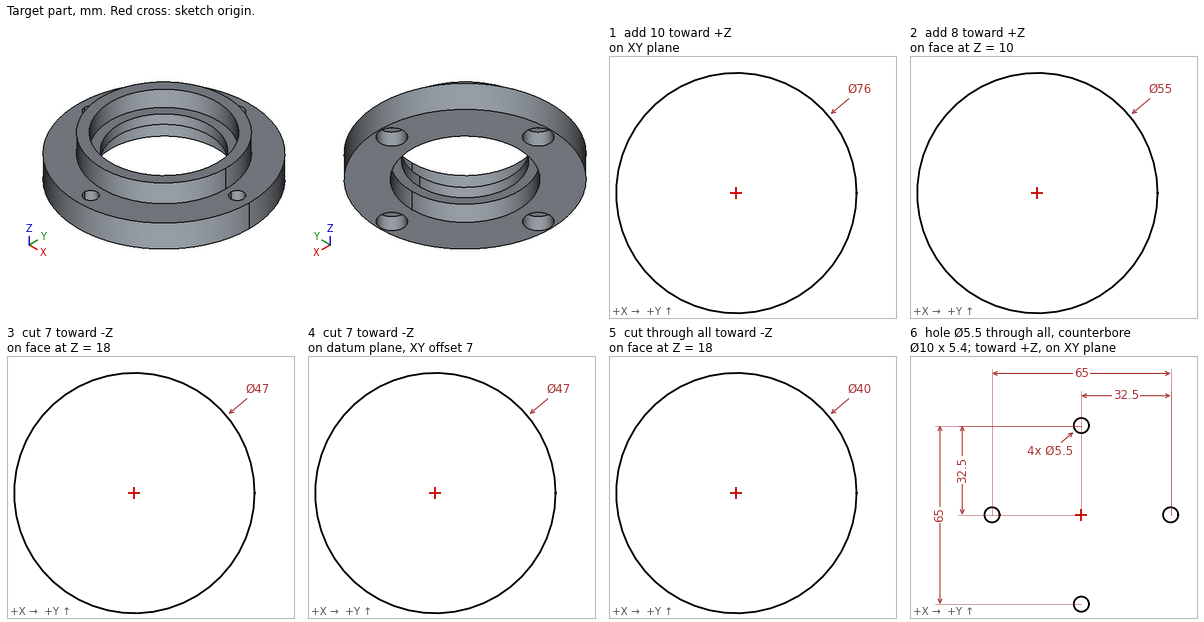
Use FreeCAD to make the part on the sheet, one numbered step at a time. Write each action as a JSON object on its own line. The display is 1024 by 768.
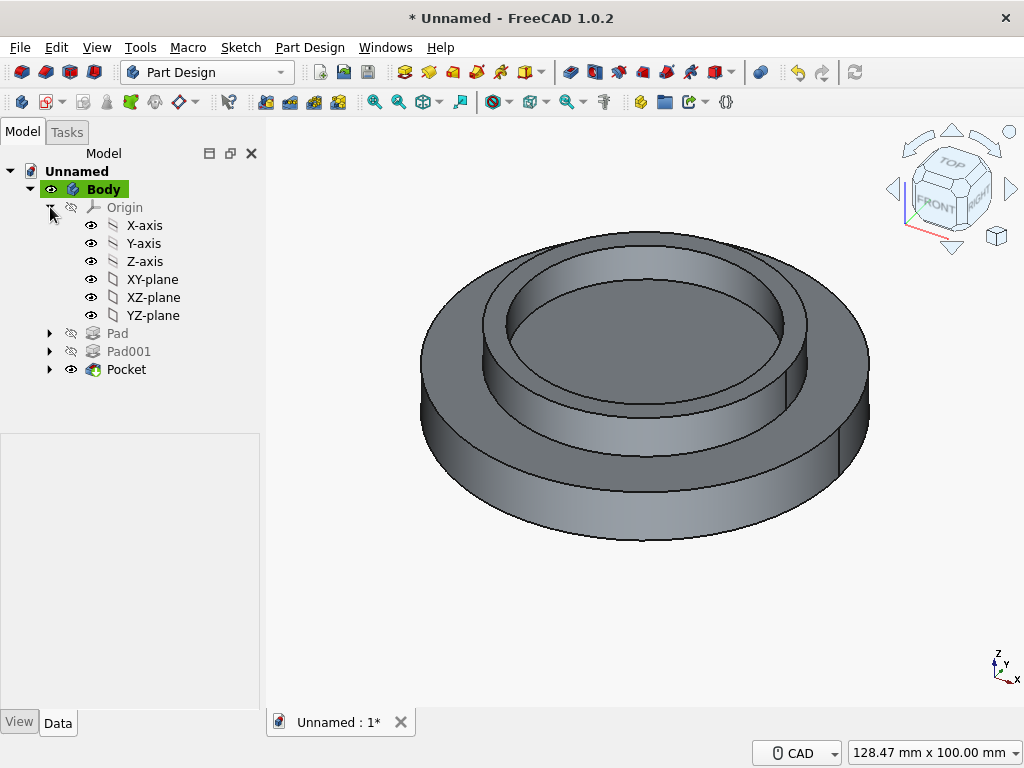
{"action": "left_click", "coordinate": [136, 279]}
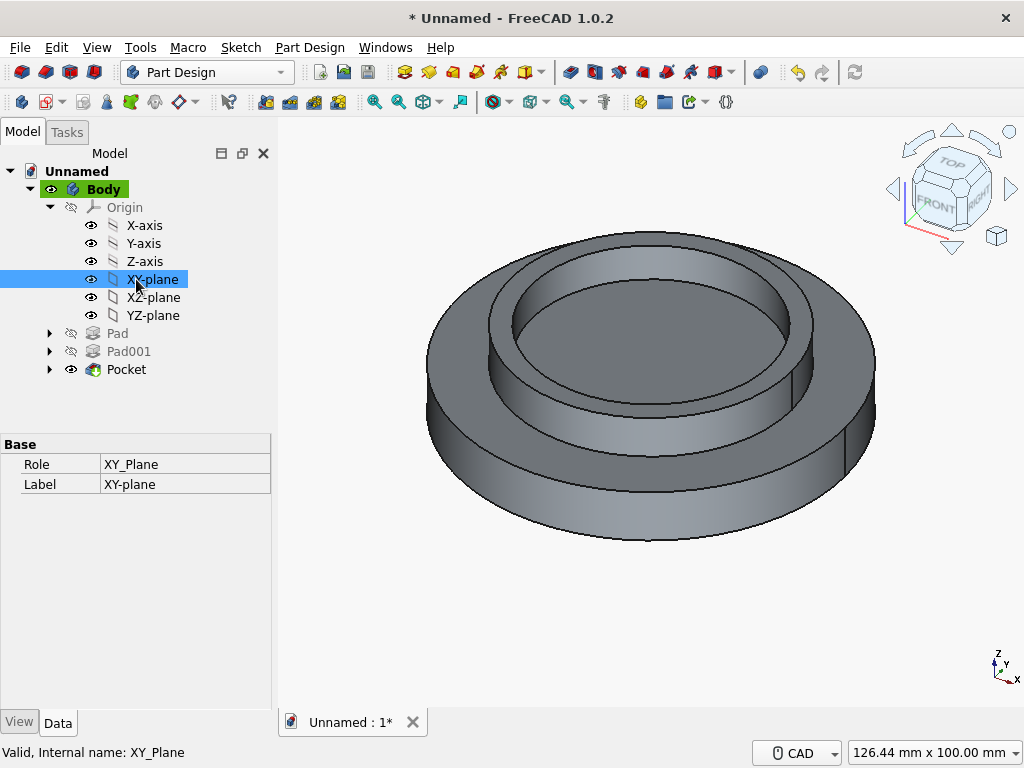
{"action": "left_click", "coordinate": [180, 102]}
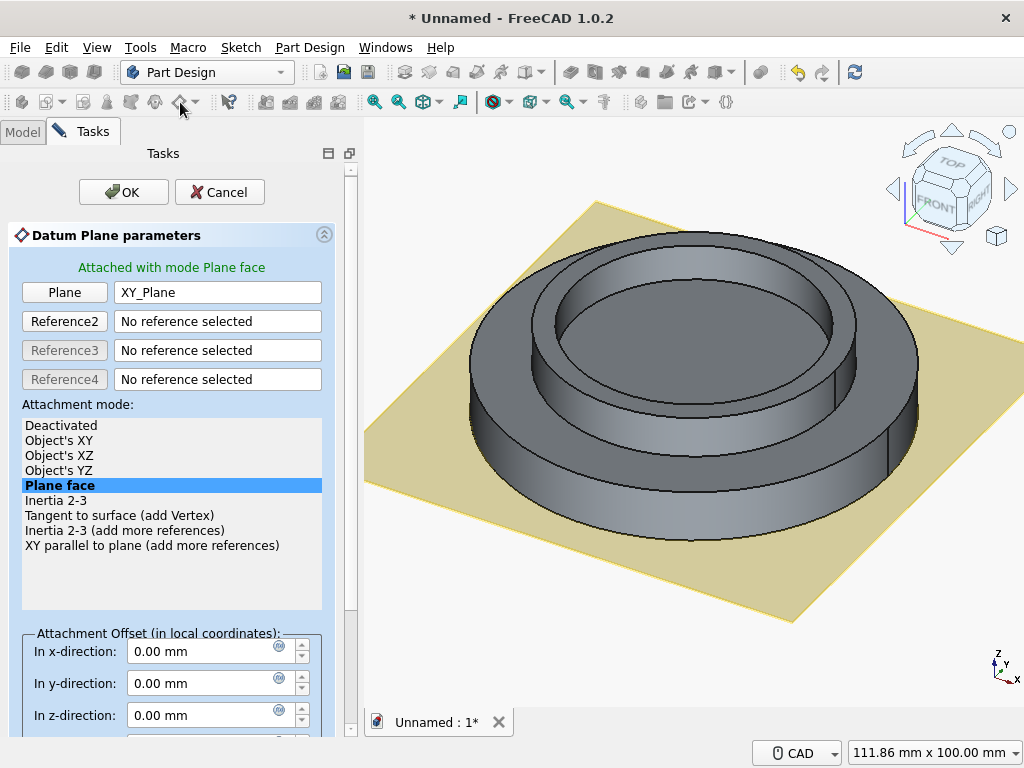
{"action": "triple_click", "coordinate": [210, 715]}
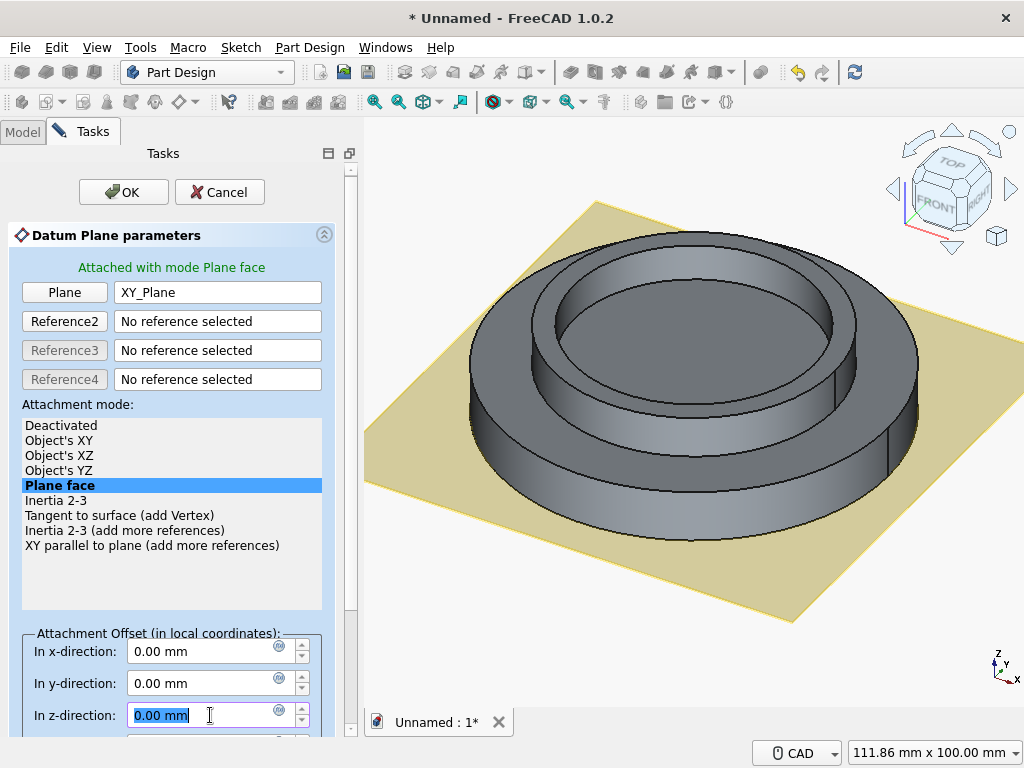
{"action": "type", "text": "7"}
{"action": "key", "text": "Tab"}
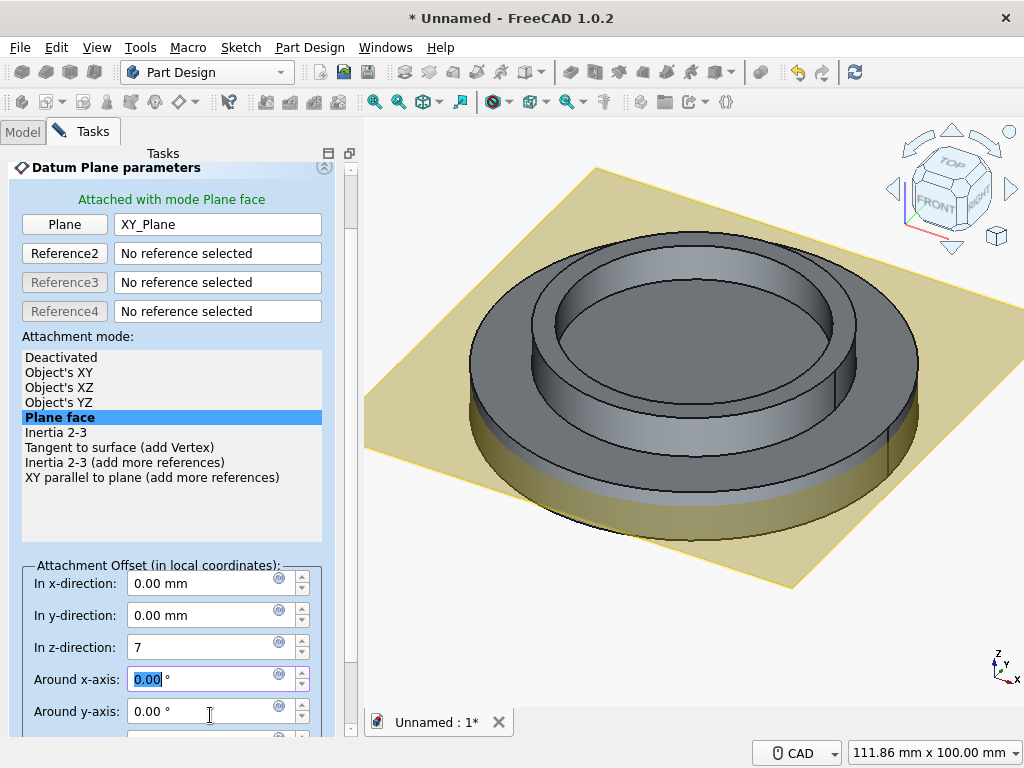
{"action": "scroll", "coordinate": [351, 450], "scroll_direction": "up", "scroll_amount": 2}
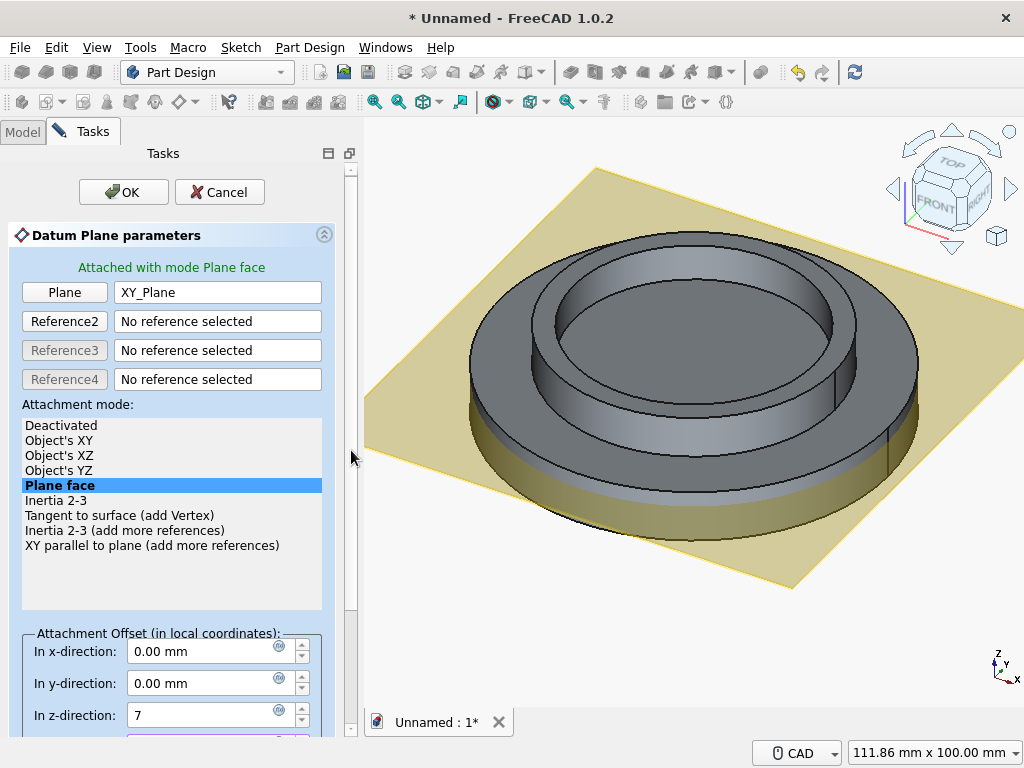
{"action": "left_click", "coordinate": [124, 192]}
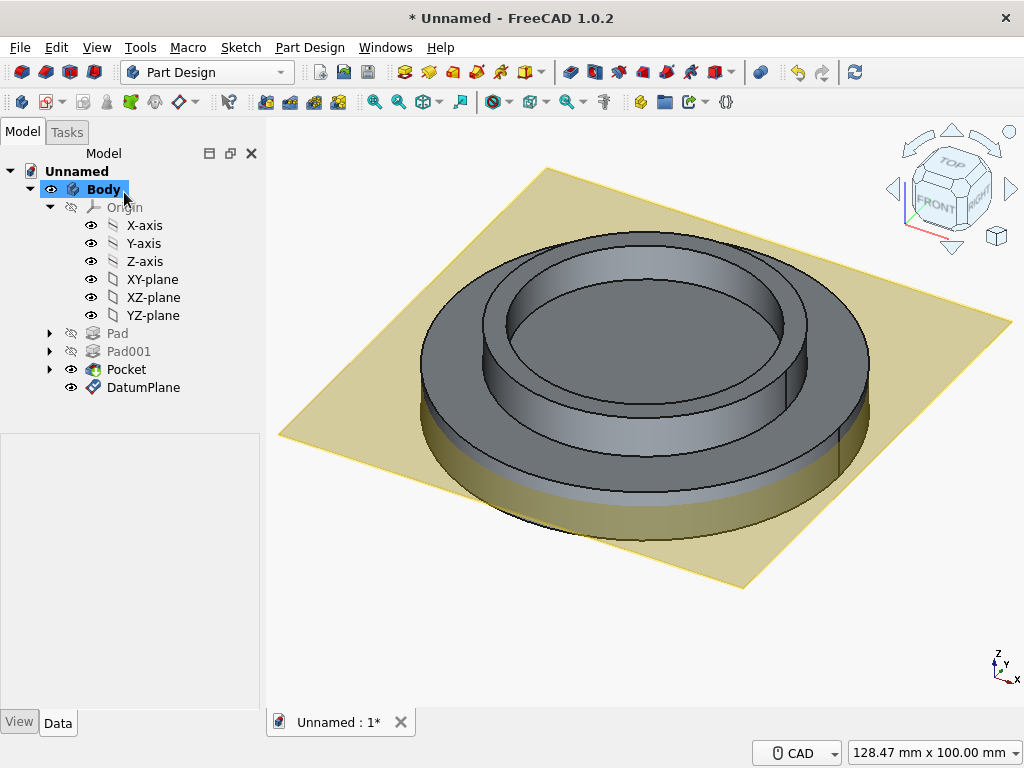
{"action": "left_click", "coordinate": [116, 387]}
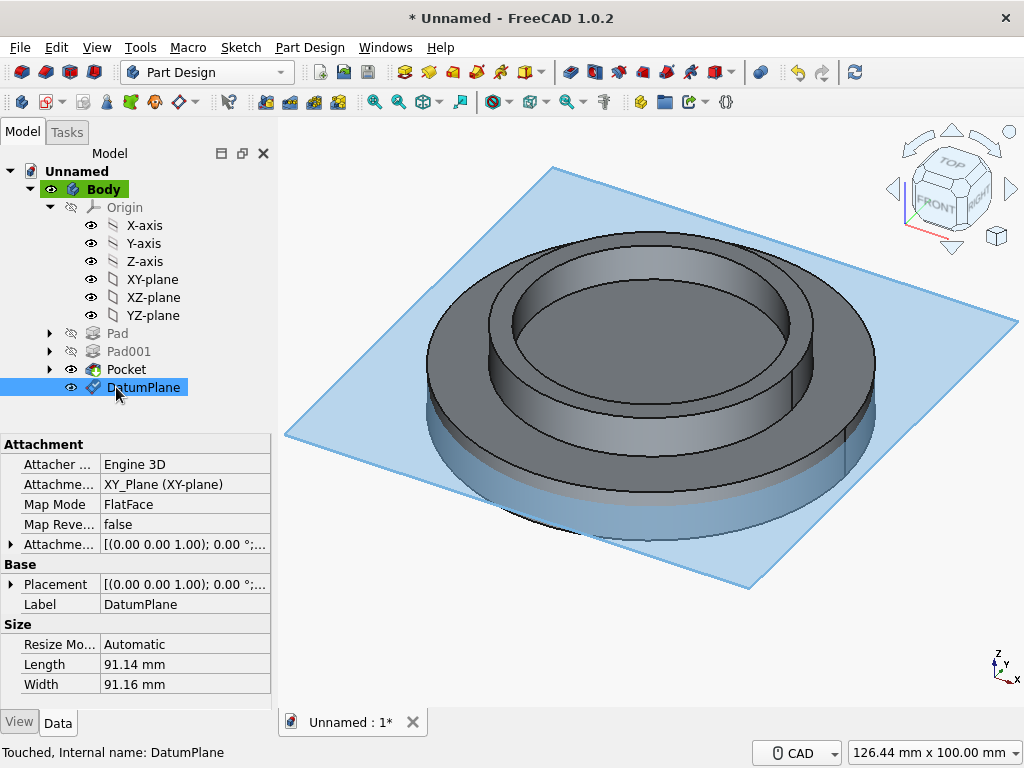
{"action": "left_click", "coordinate": [46, 102]}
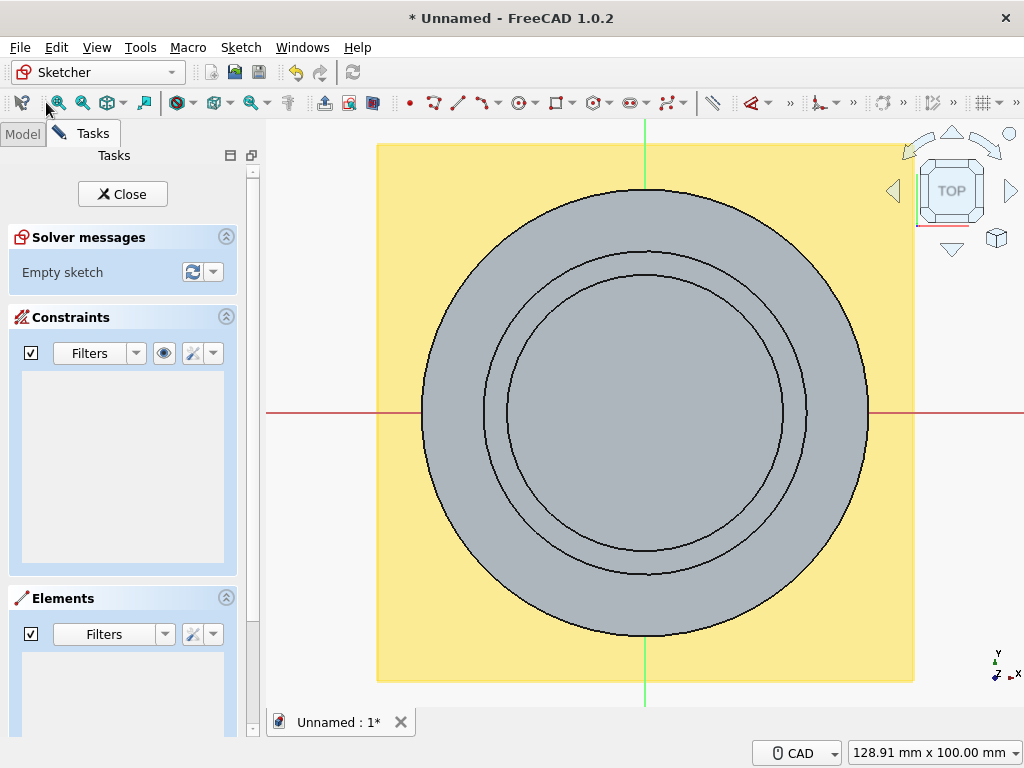
{"action": "left_click", "coordinate": [374, 104]}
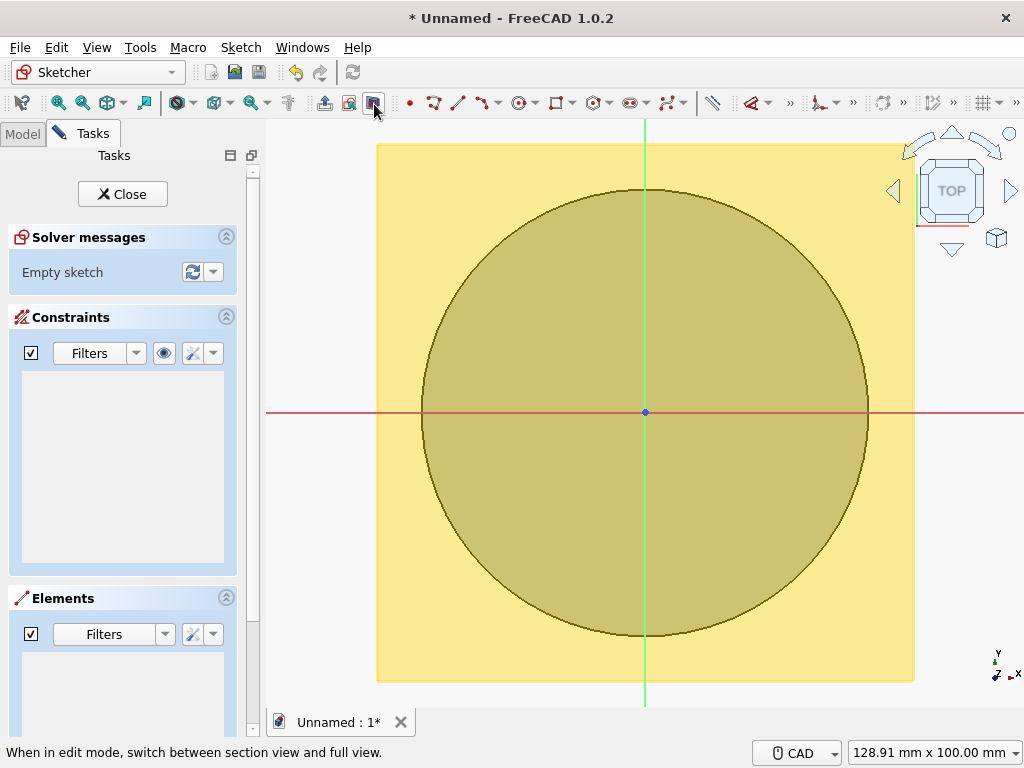
{"action": "scroll", "coordinate": [784, 413], "scroll_direction": "up", "scroll_amount": 2}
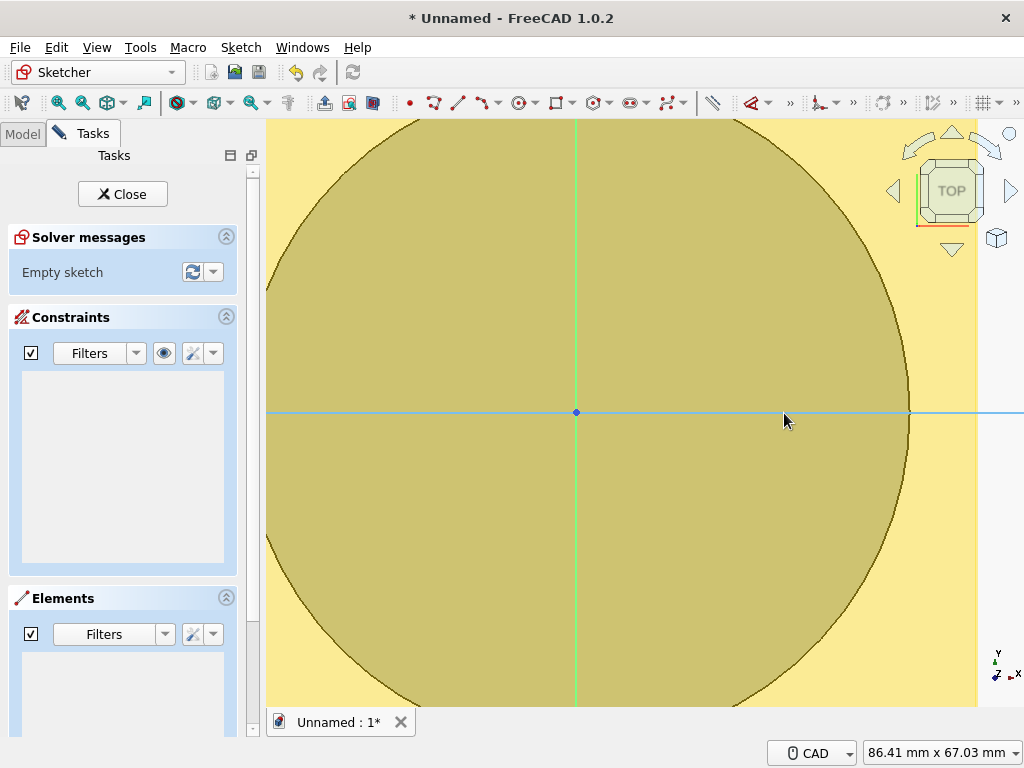
{"action": "key", "text": "g c"}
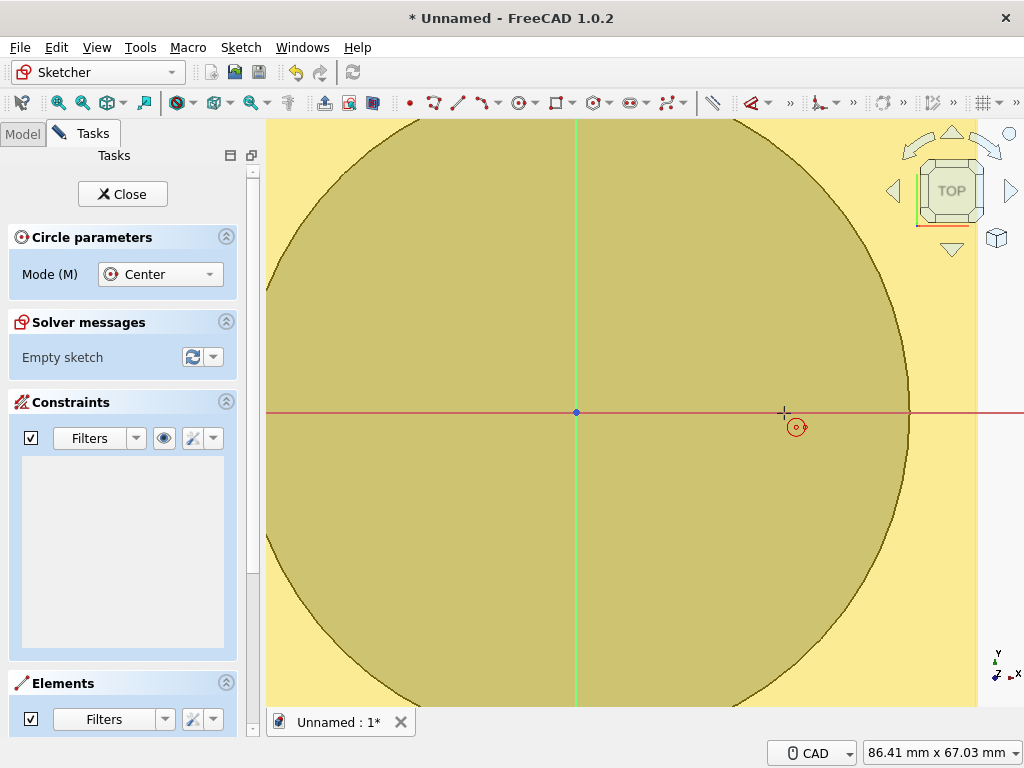
{"action": "left_click", "coordinate": [576, 413]}
{"action": "left_click", "coordinate": [722, 267]}
{"action": "key", "text": "Escape"}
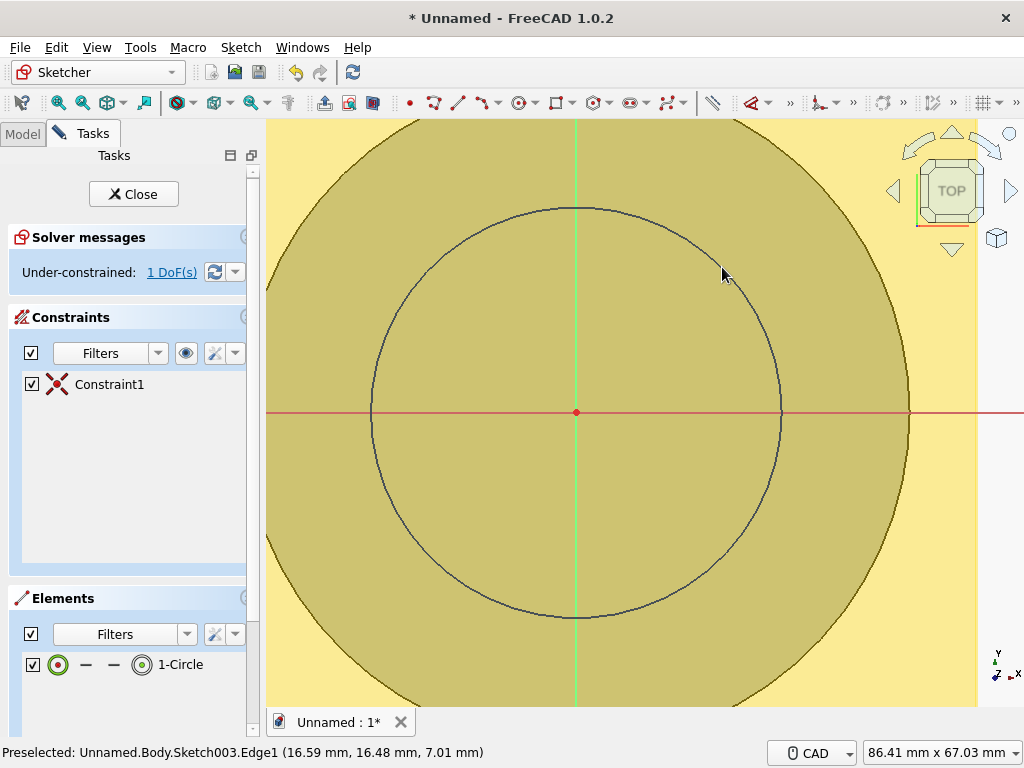
{"action": "left_click", "coordinate": [721, 267]}